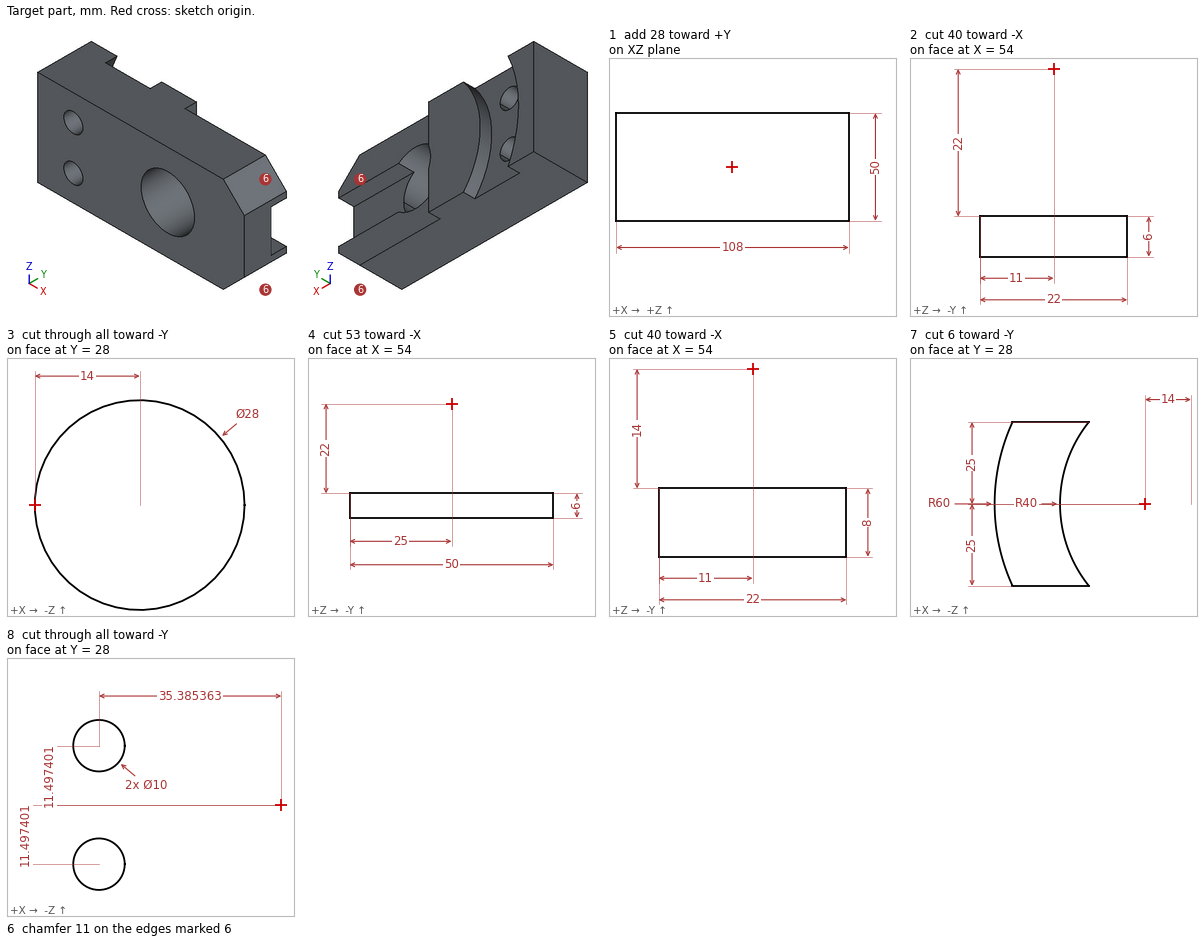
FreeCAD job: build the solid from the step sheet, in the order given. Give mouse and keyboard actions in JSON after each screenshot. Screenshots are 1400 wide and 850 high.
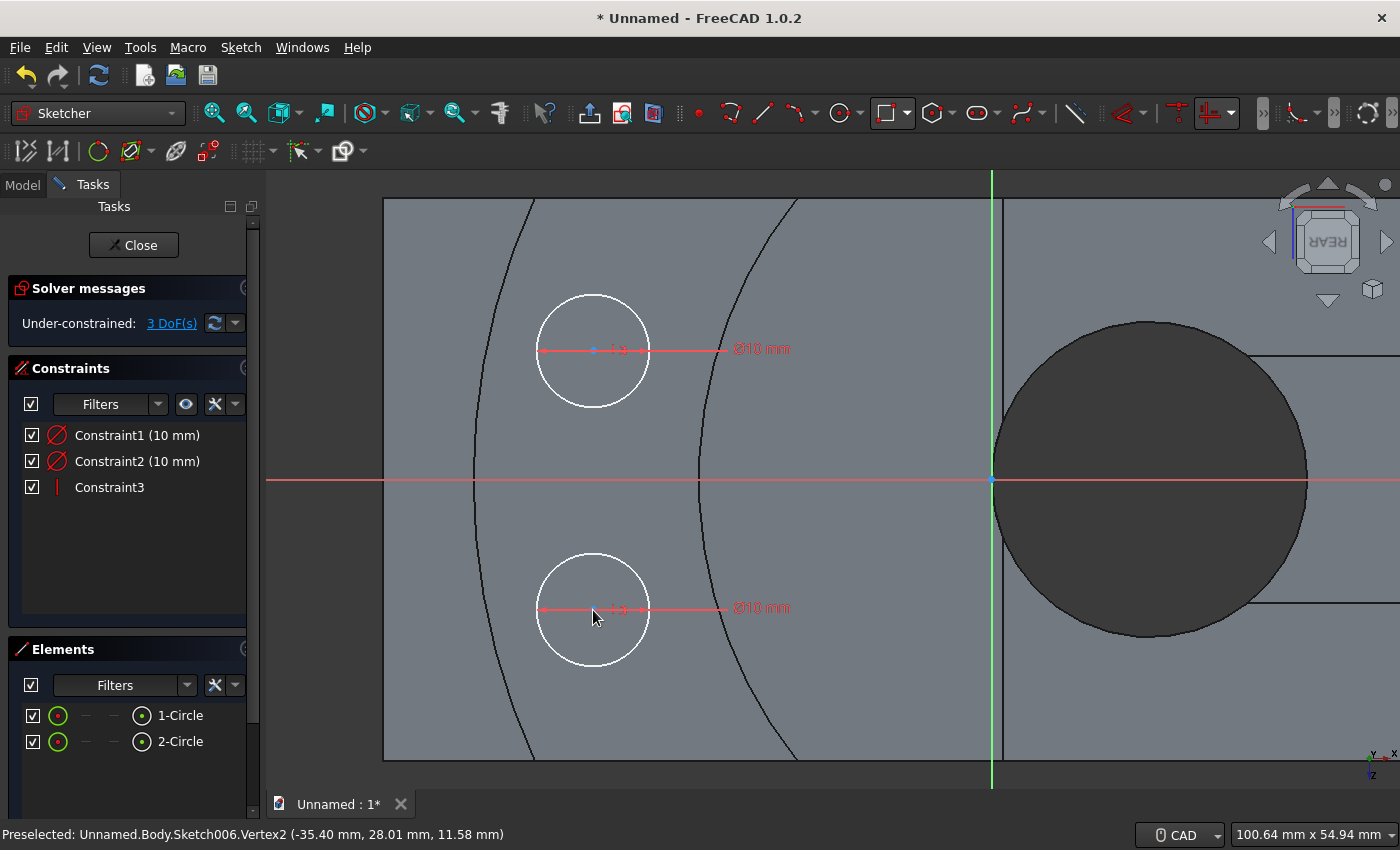
{"action": "key", "text": "d"}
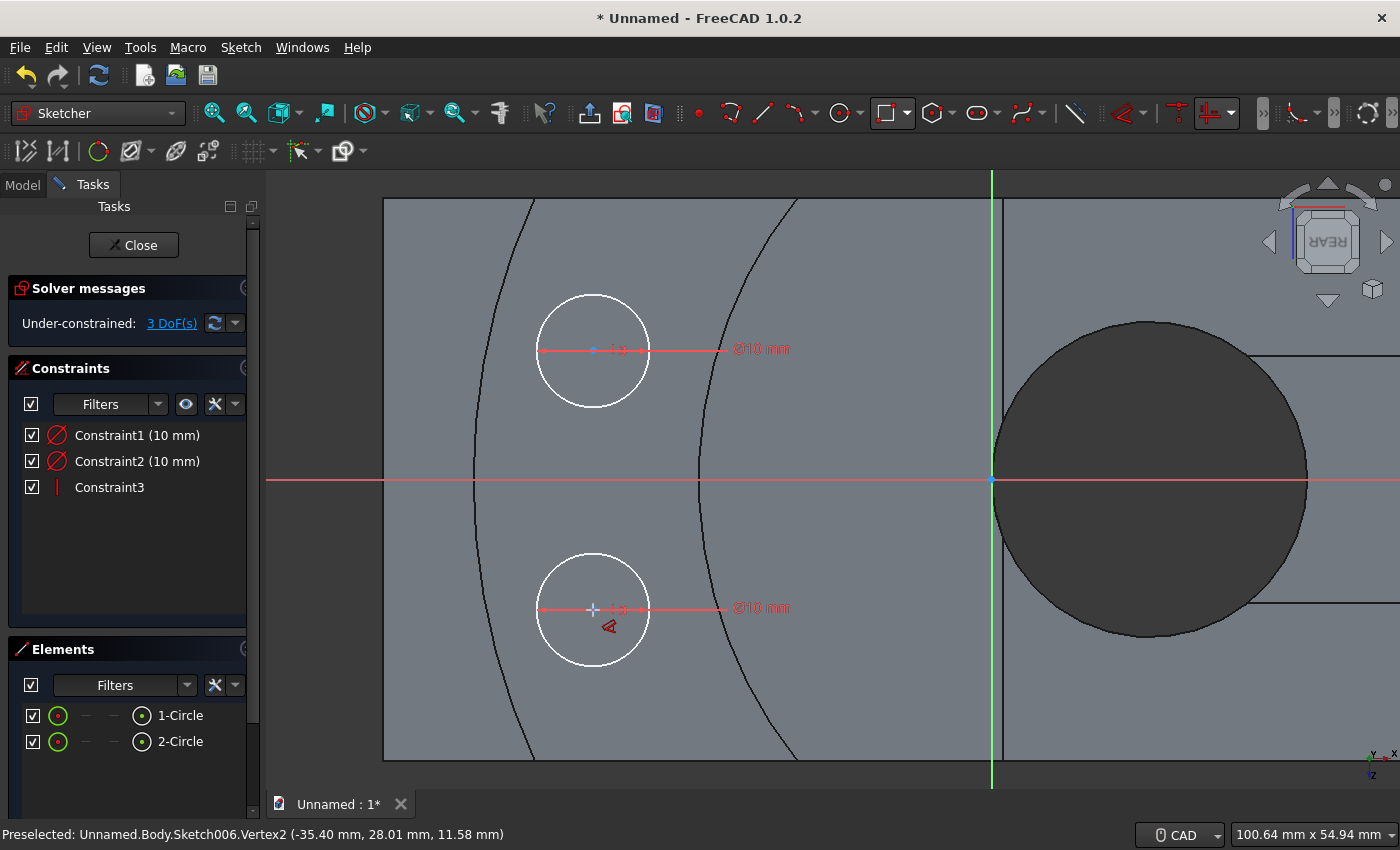
{"action": "left_click", "coordinate": [593, 351]}
{"action": "left_click", "coordinate": [792, 317]}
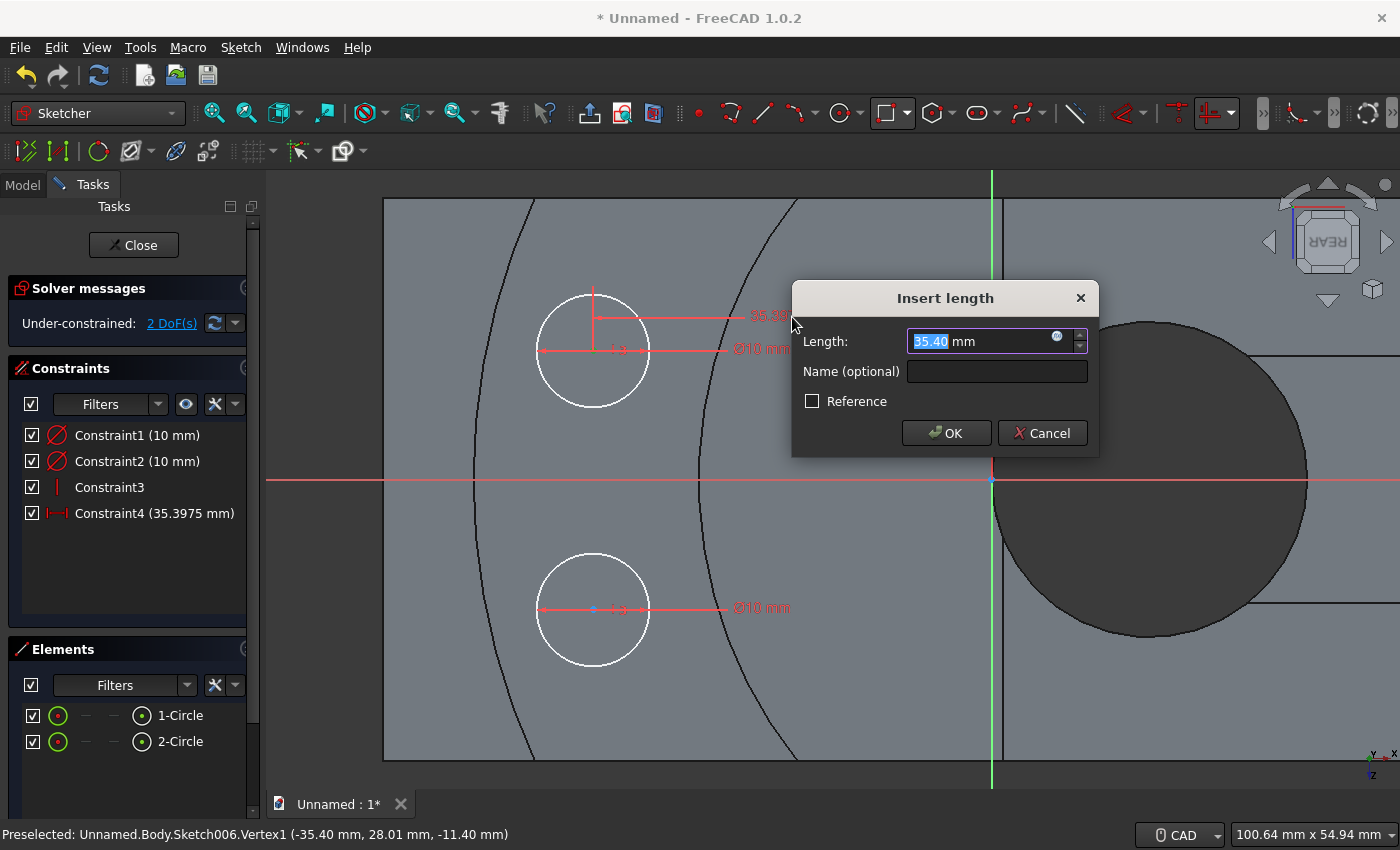
{"action": "type", "text": "35.385363"}
{"action": "key", "text": "Return"}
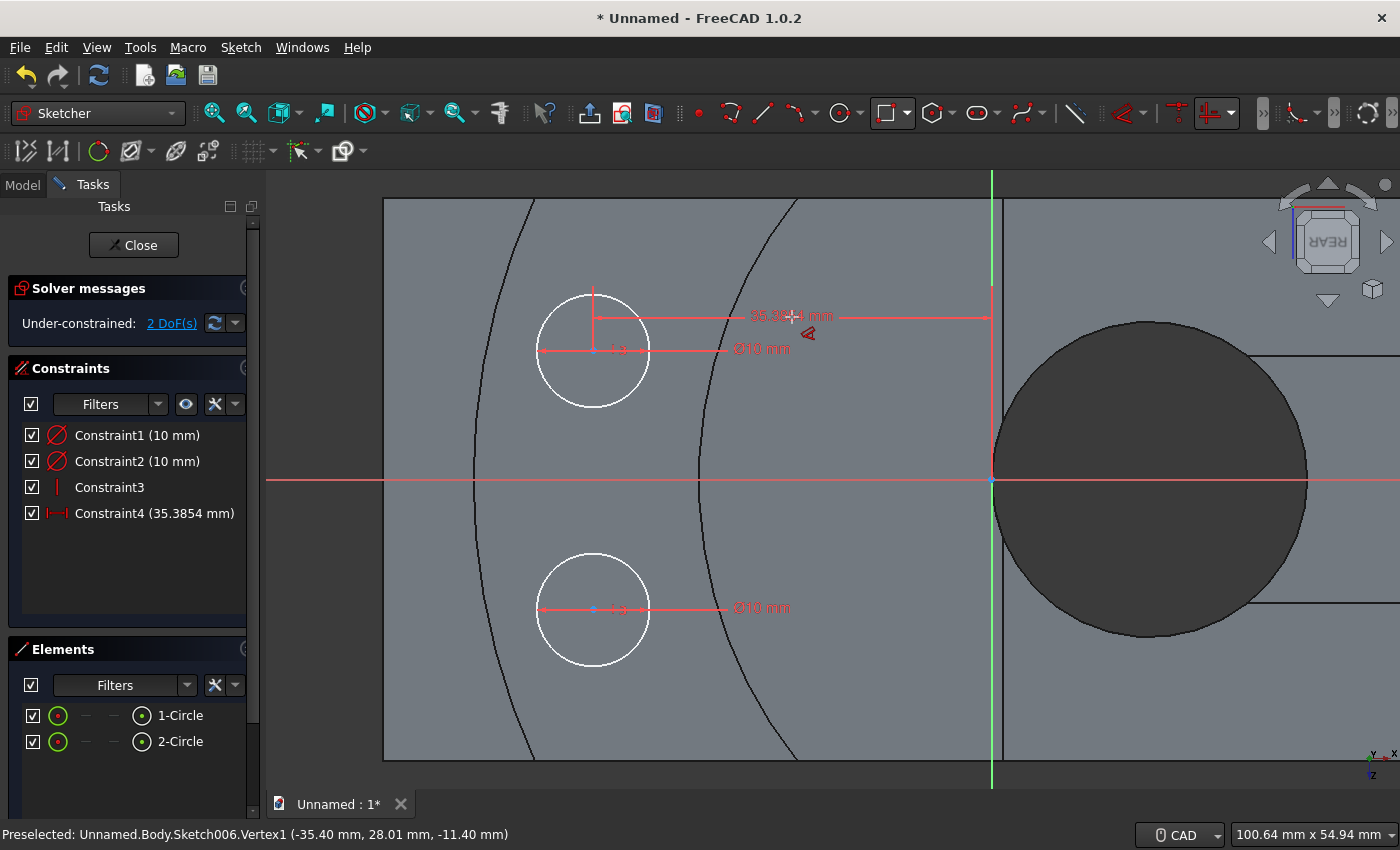
{"action": "left_click", "coordinate": [593, 351]}
{"action": "left_click", "coordinate": [1026, 415]}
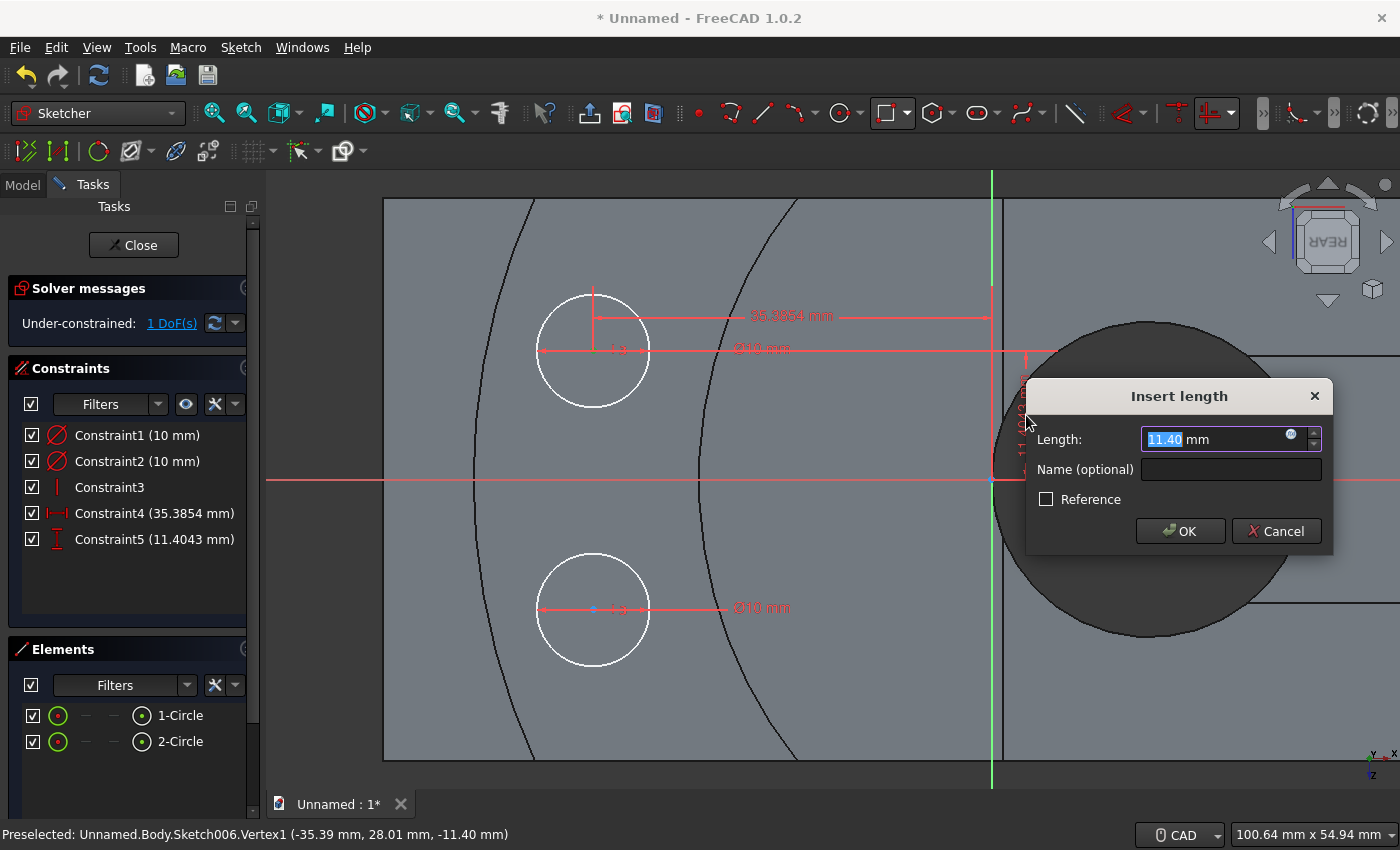
{"action": "type", "text": "11.497401"}
{"action": "key", "text": "Return"}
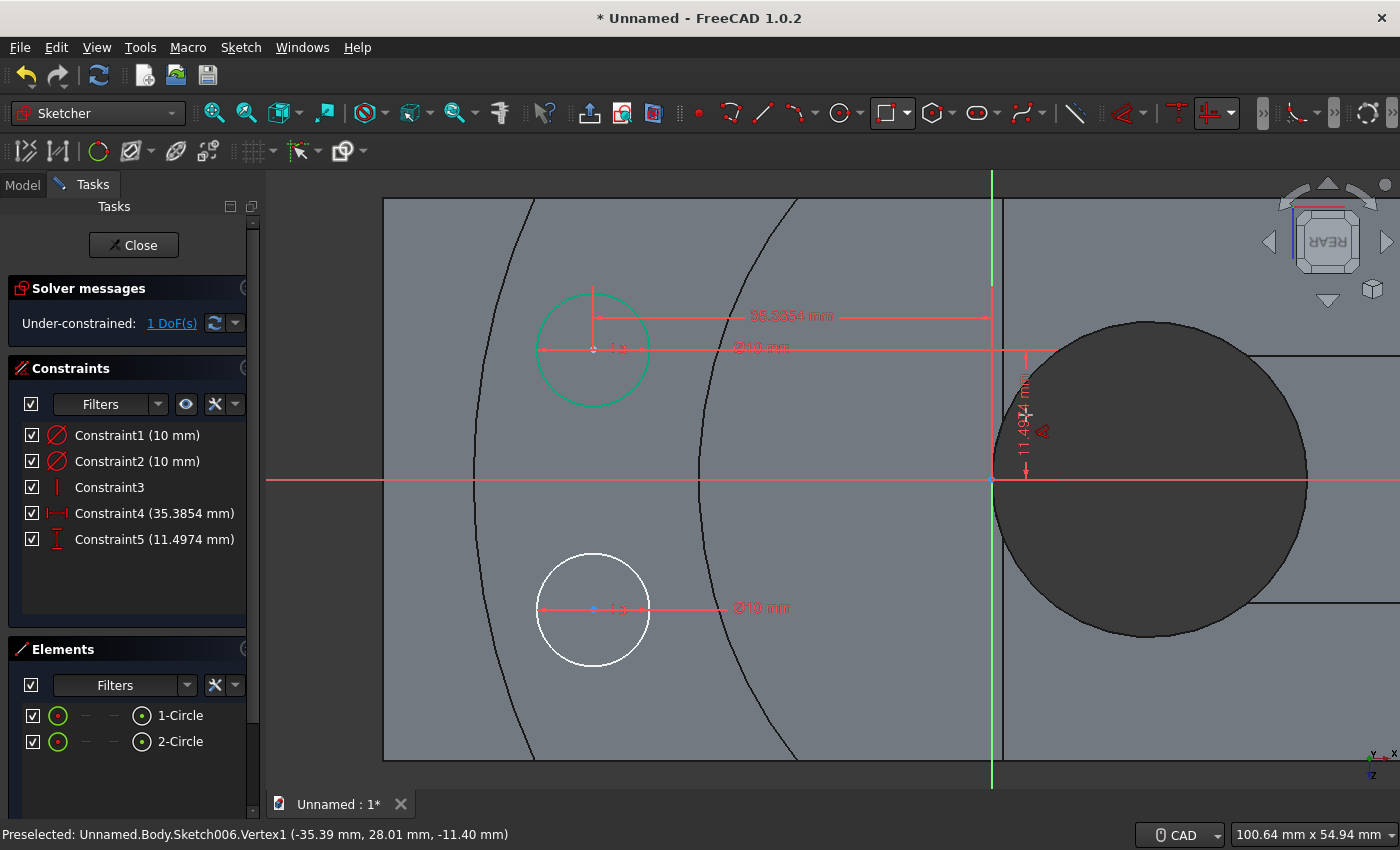
{"action": "left_click", "coordinate": [593, 610]}
{"action": "left_click", "coordinate": [1026, 545]}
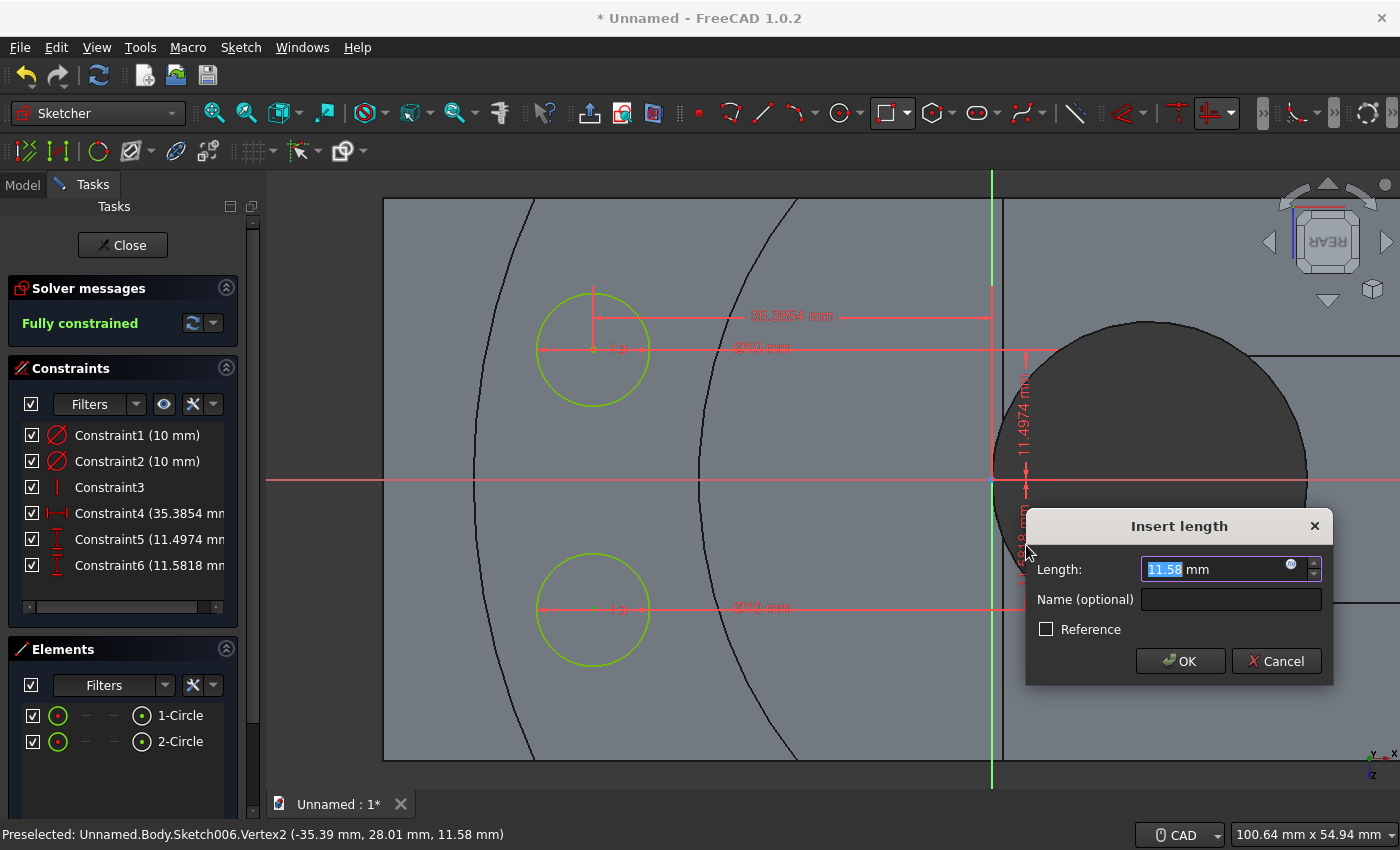
{"action": "type", "text": "11.497401"}
{"action": "key", "text": "Return"}
{"action": "key", "text": "Escape"}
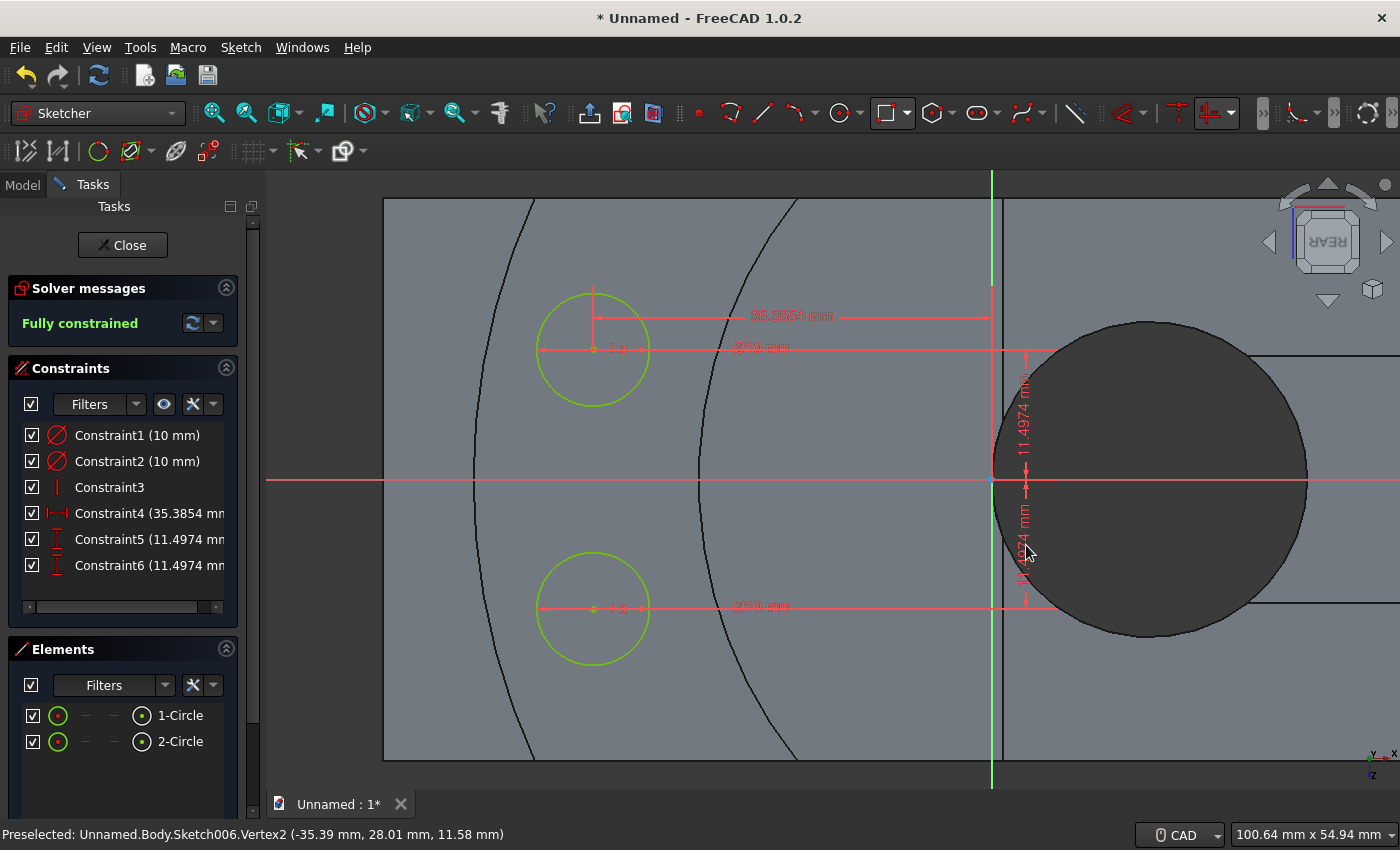
{"action": "left_click", "coordinate": [123, 245]}